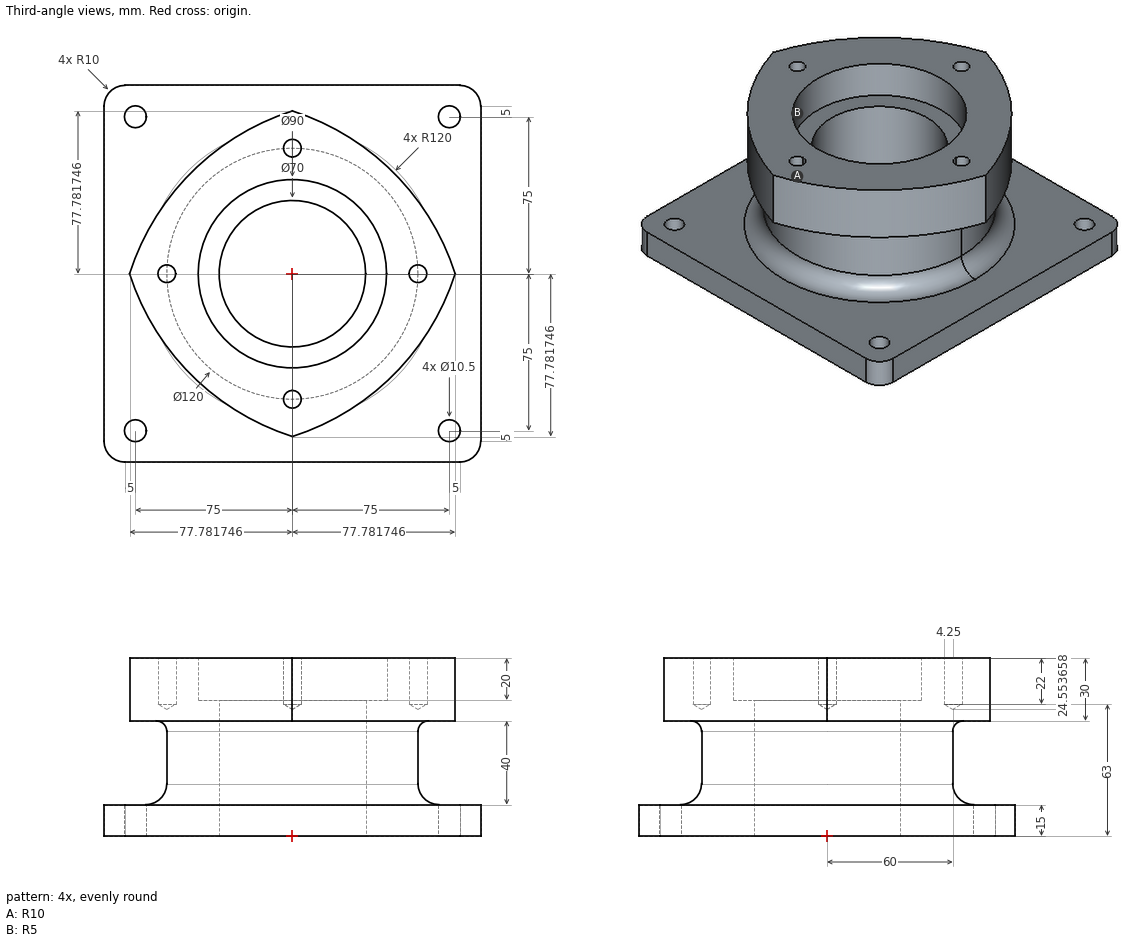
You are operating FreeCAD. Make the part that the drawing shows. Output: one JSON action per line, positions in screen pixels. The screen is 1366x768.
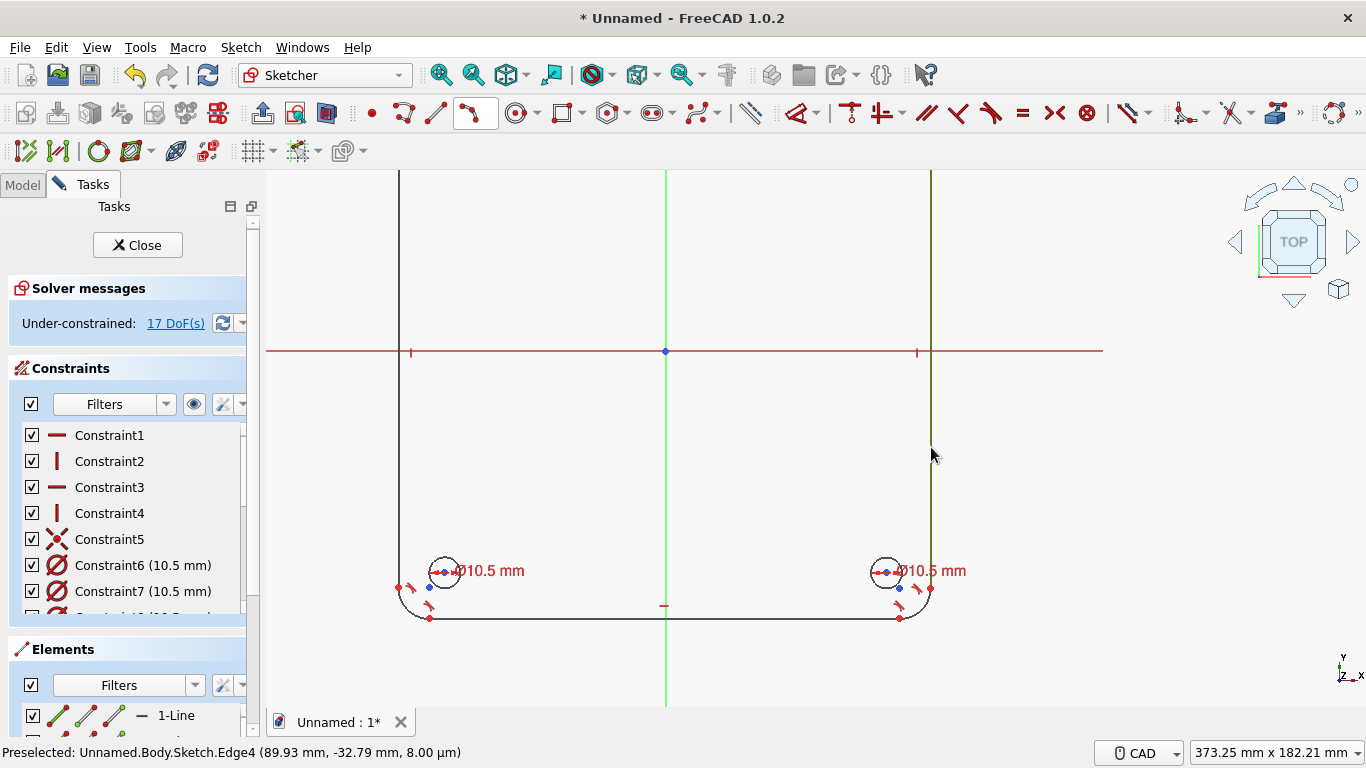
{"action": "scroll", "coordinate": [914, 616], "scroll_direction": "down", "scroll_amount": 2}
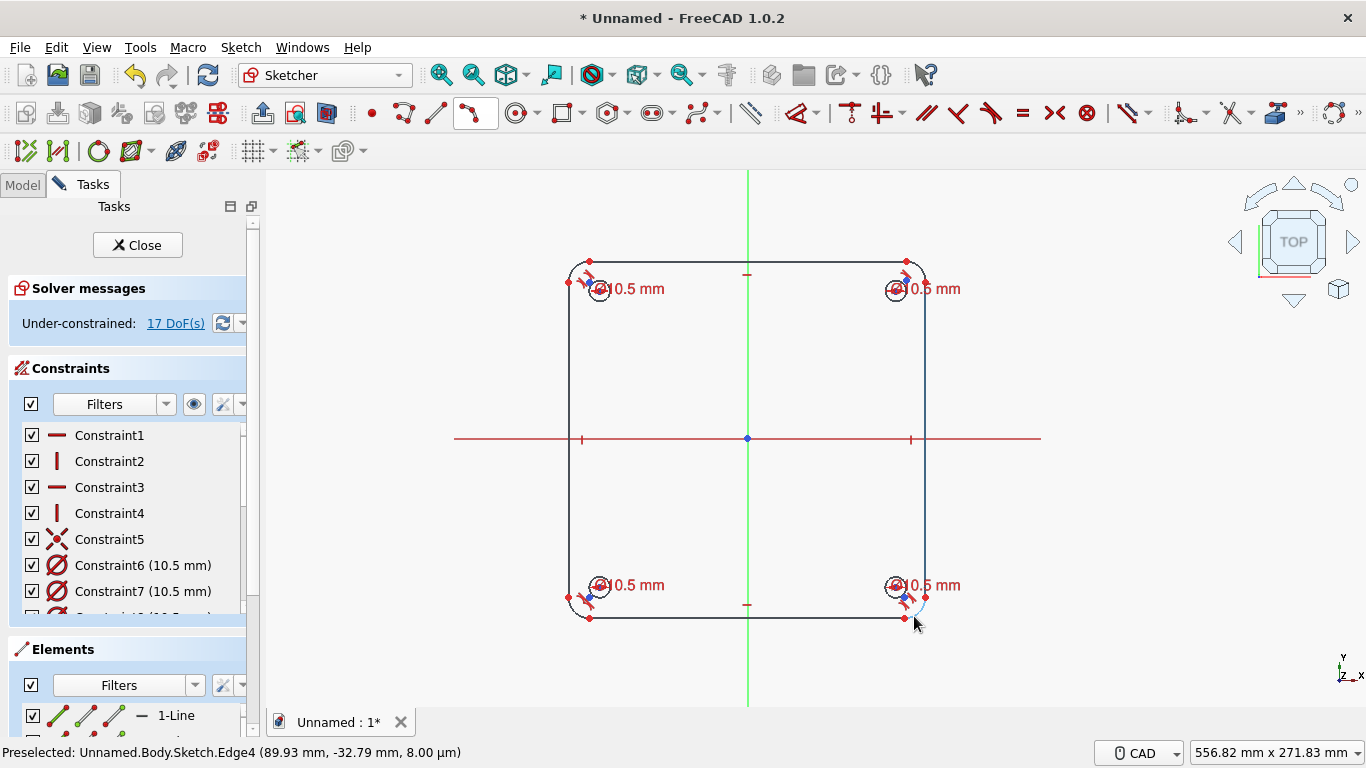
{"action": "scroll", "coordinate": [924, 273], "scroll_direction": "up", "scroll_amount": 2}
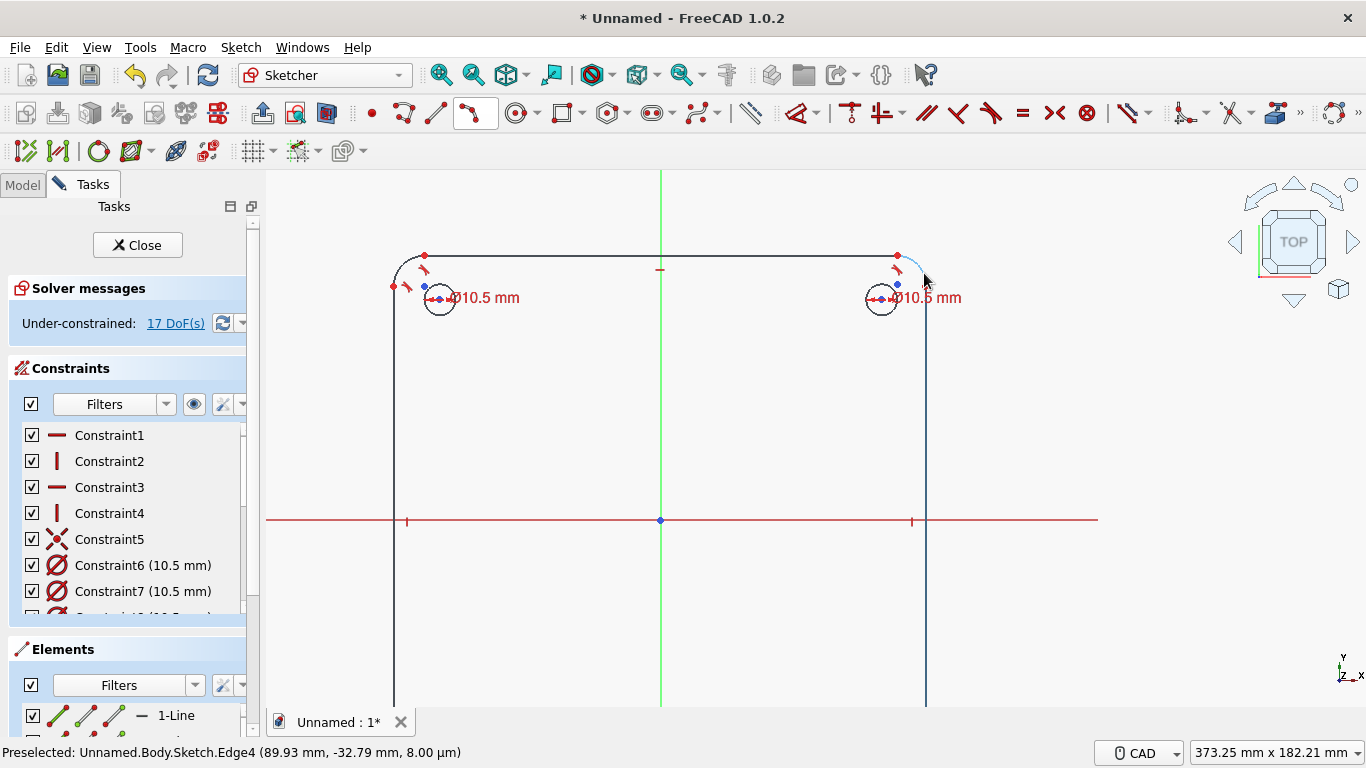
{"action": "left_click", "coordinate": [923, 273]}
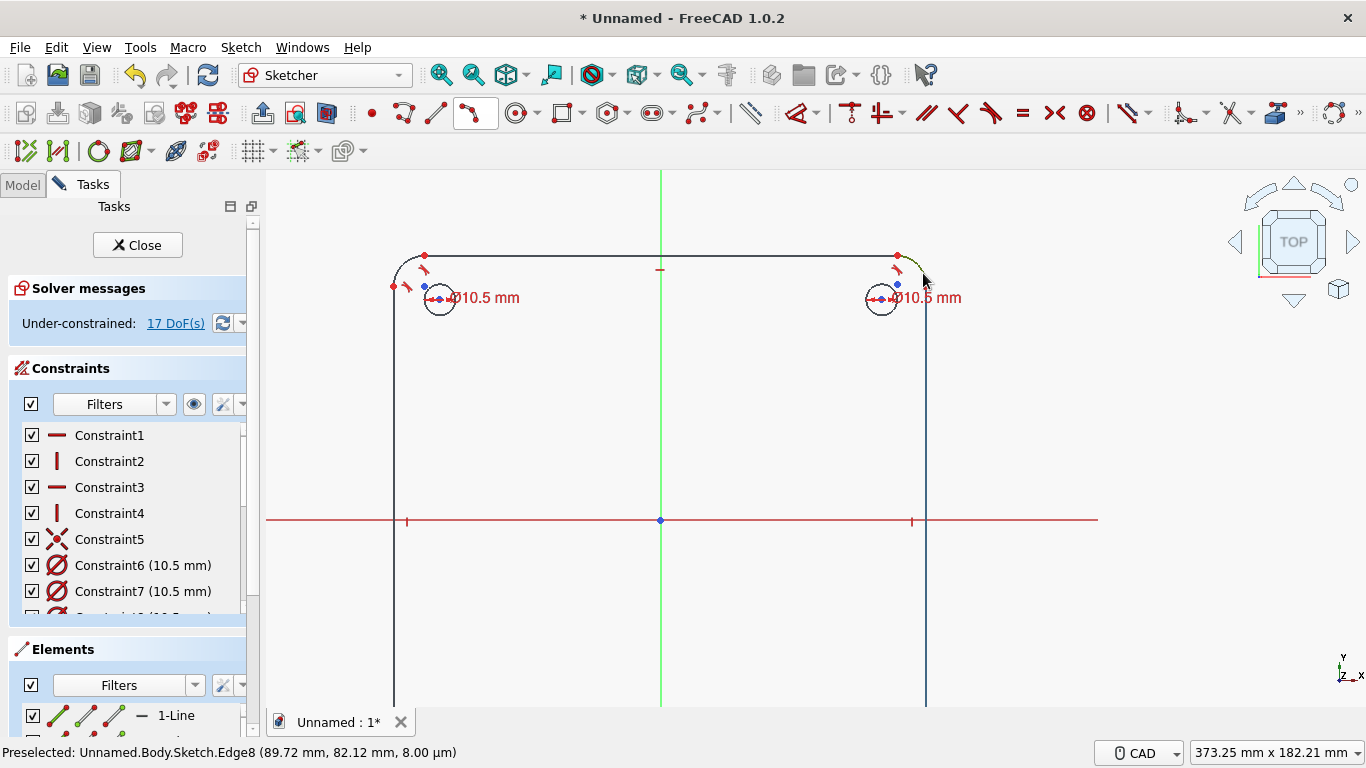
{"action": "left_click", "coordinate": [992, 114]}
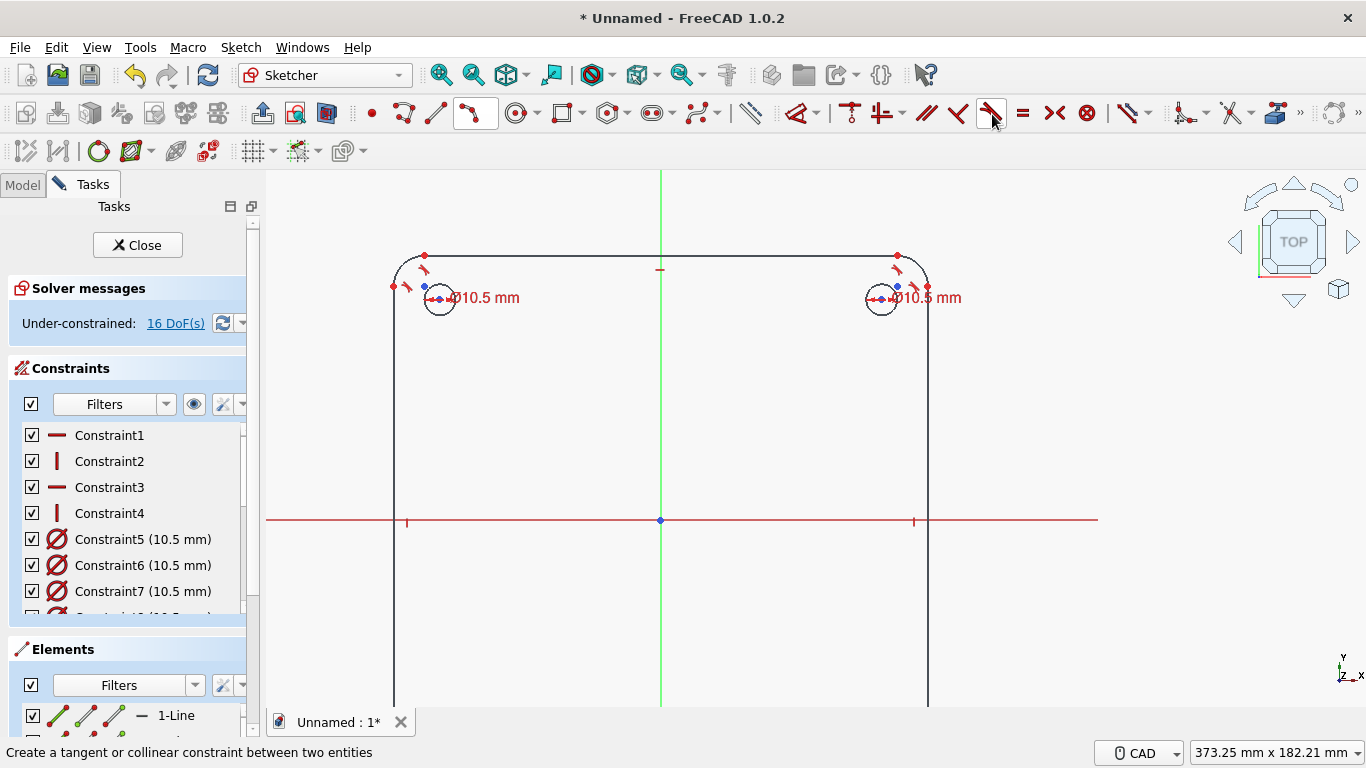
{"action": "left_click", "coordinate": [411, 259]}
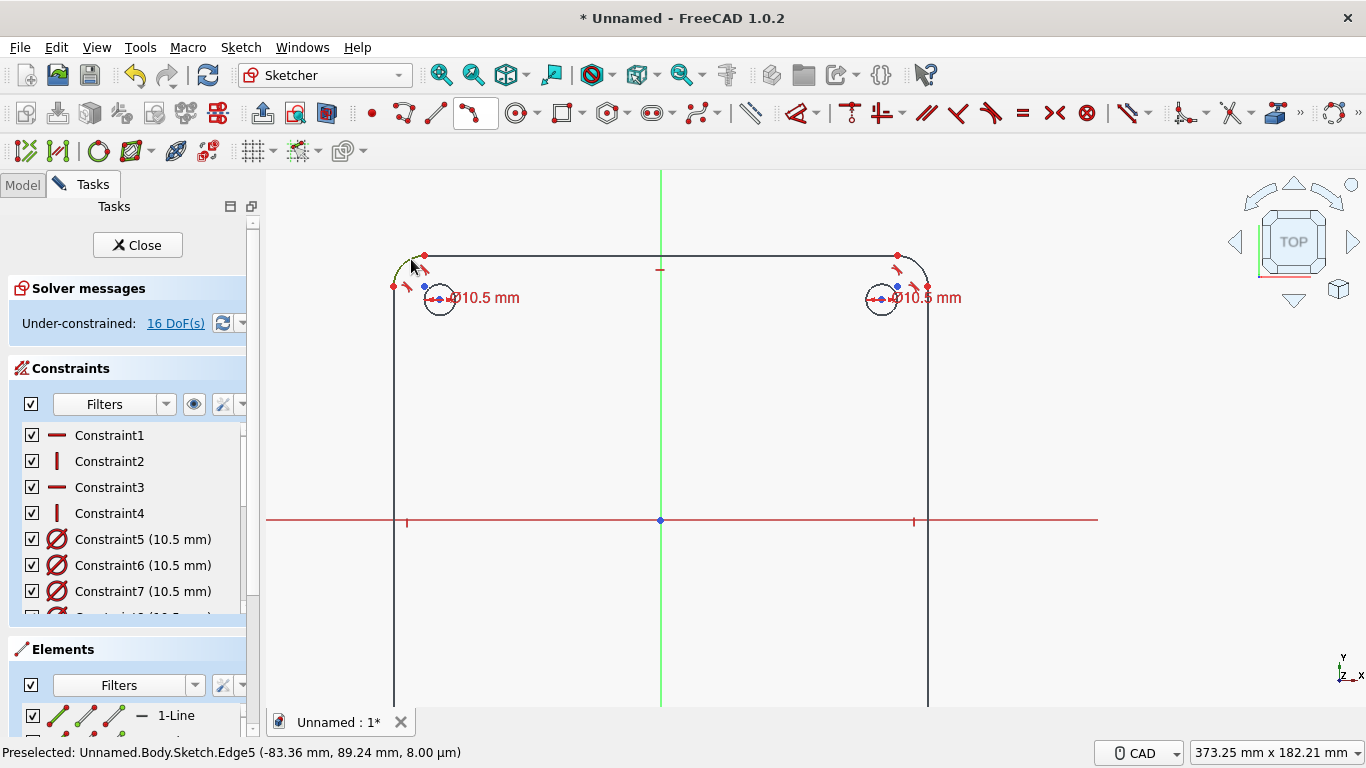
{"action": "scroll", "coordinate": [924, 272], "scroll_direction": "down", "scroll_amount": 2}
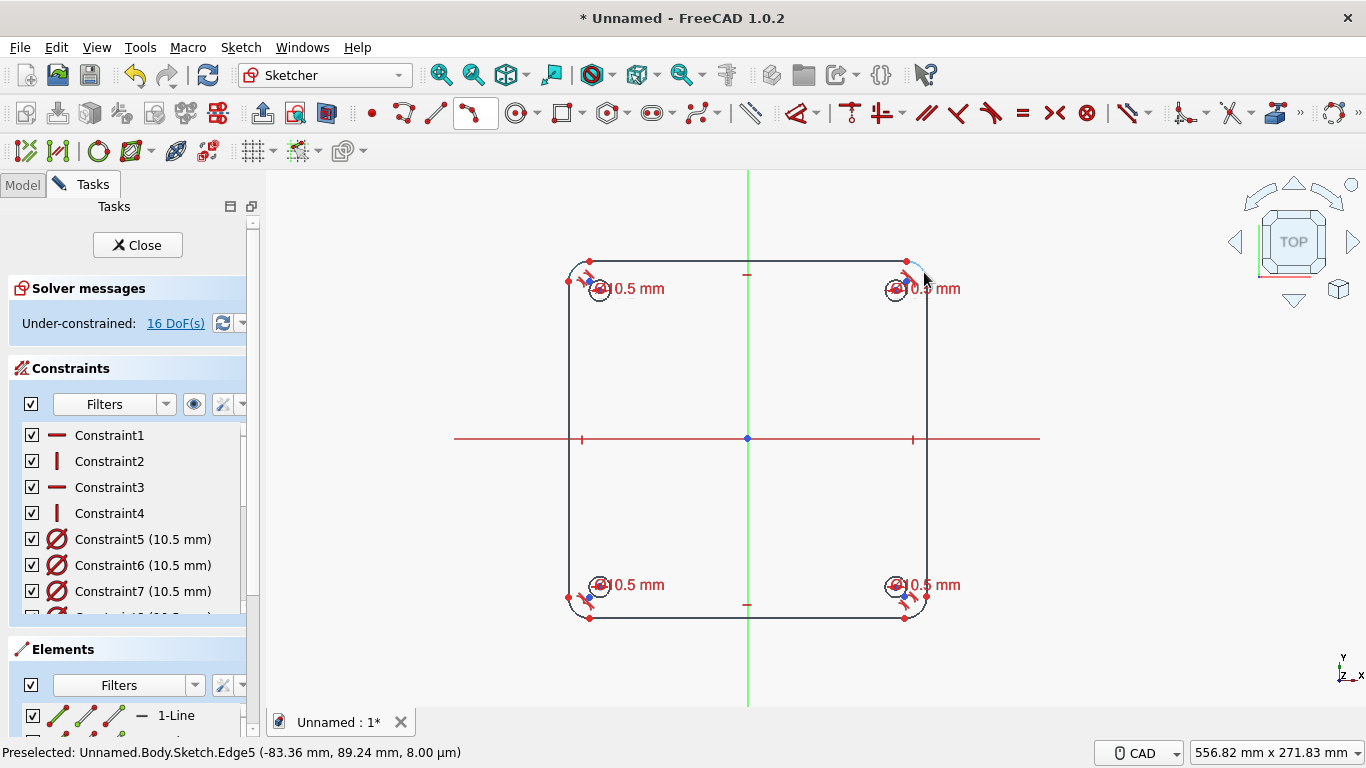
{"action": "scroll", "coordinate": [571, 607], "scroll_direction": "up", "scroll_amount": 2}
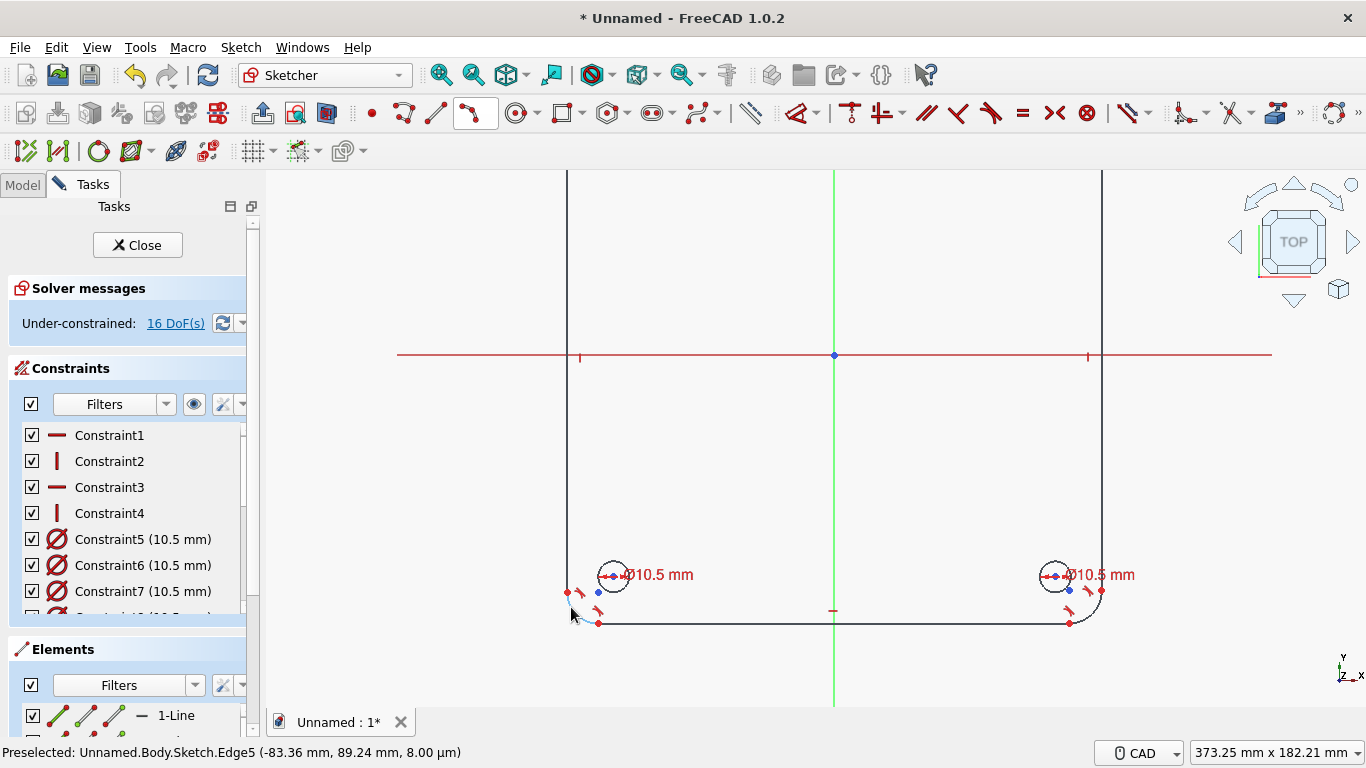
{"action": "left_click", "coordinate": [571, 607]}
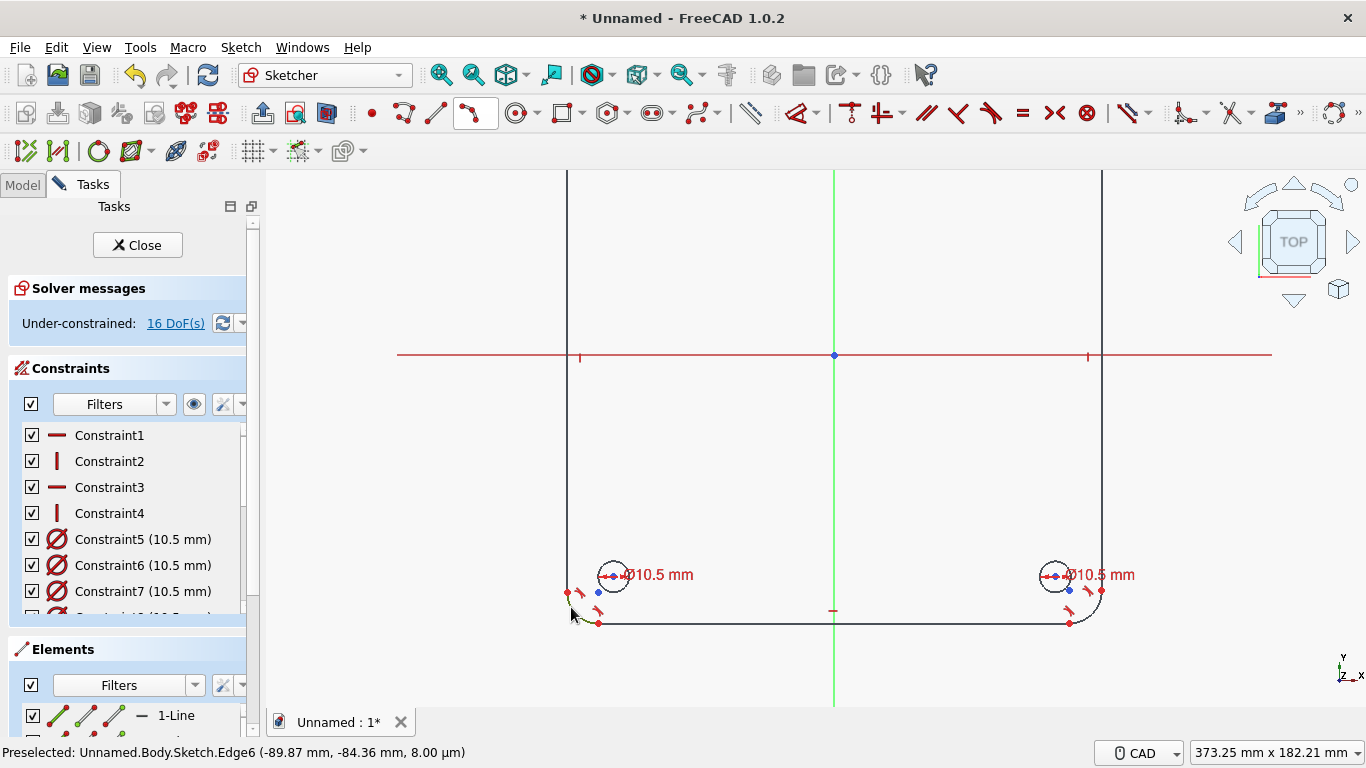
{"action": "left_click", "coordinate": [1084, 620]}